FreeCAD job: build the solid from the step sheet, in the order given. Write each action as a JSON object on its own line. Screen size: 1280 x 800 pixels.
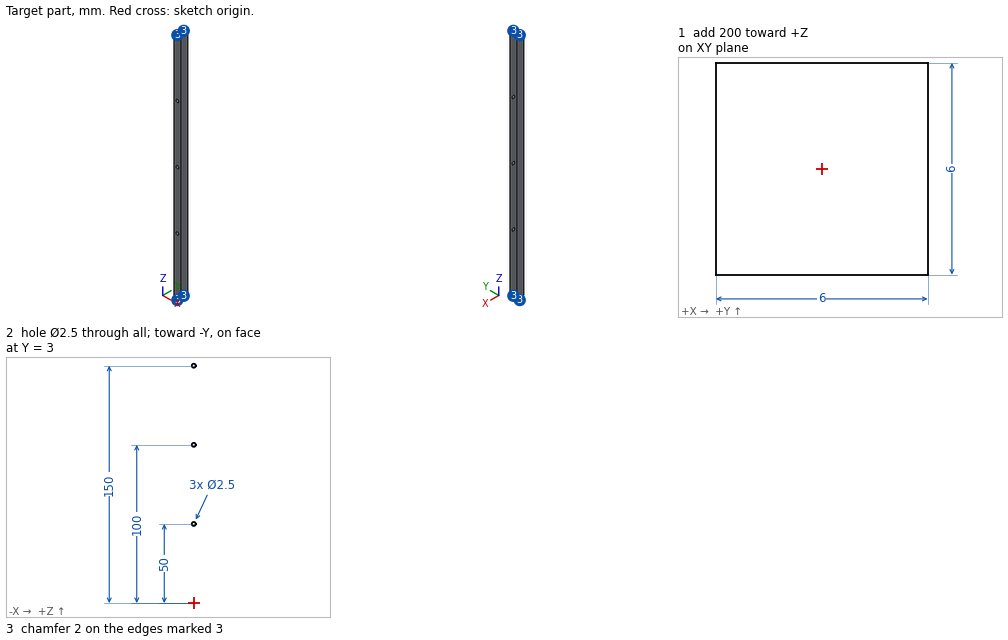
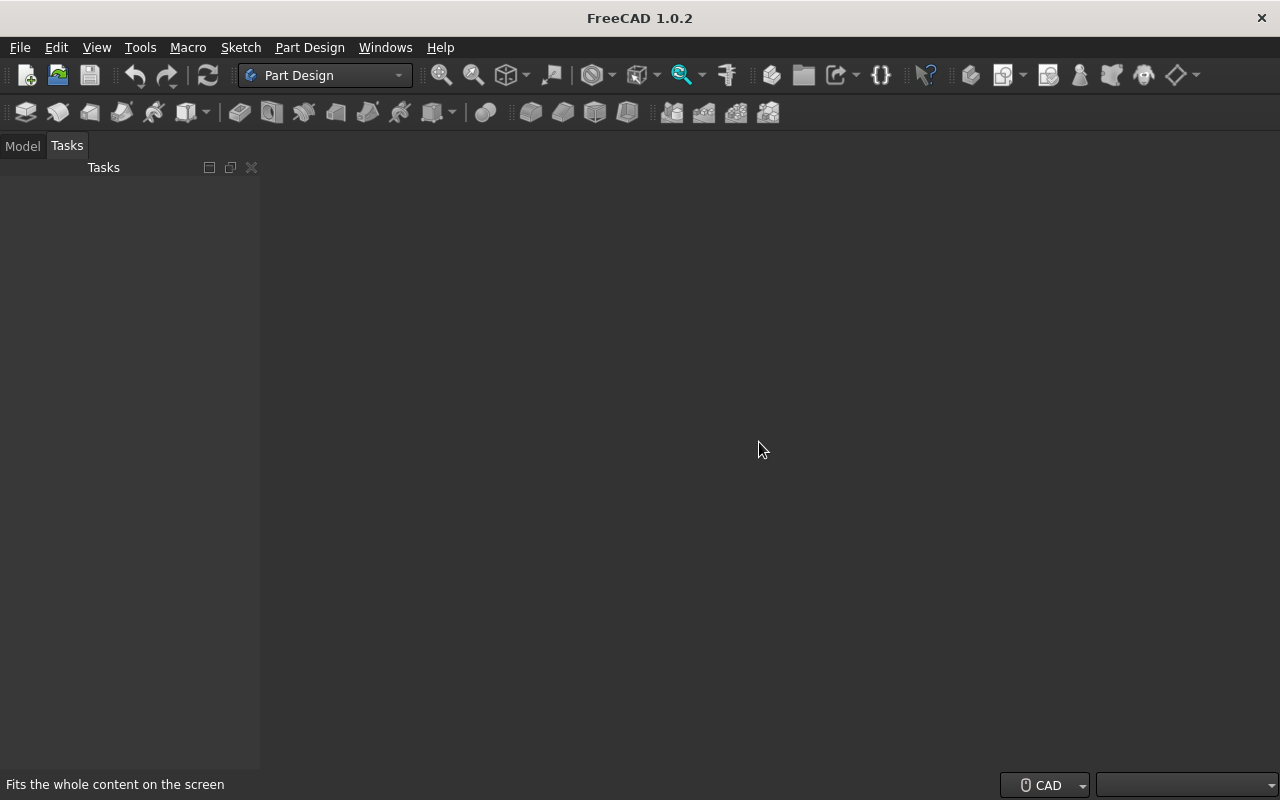
{"action": "left_click", "coordinate": [26, 76]}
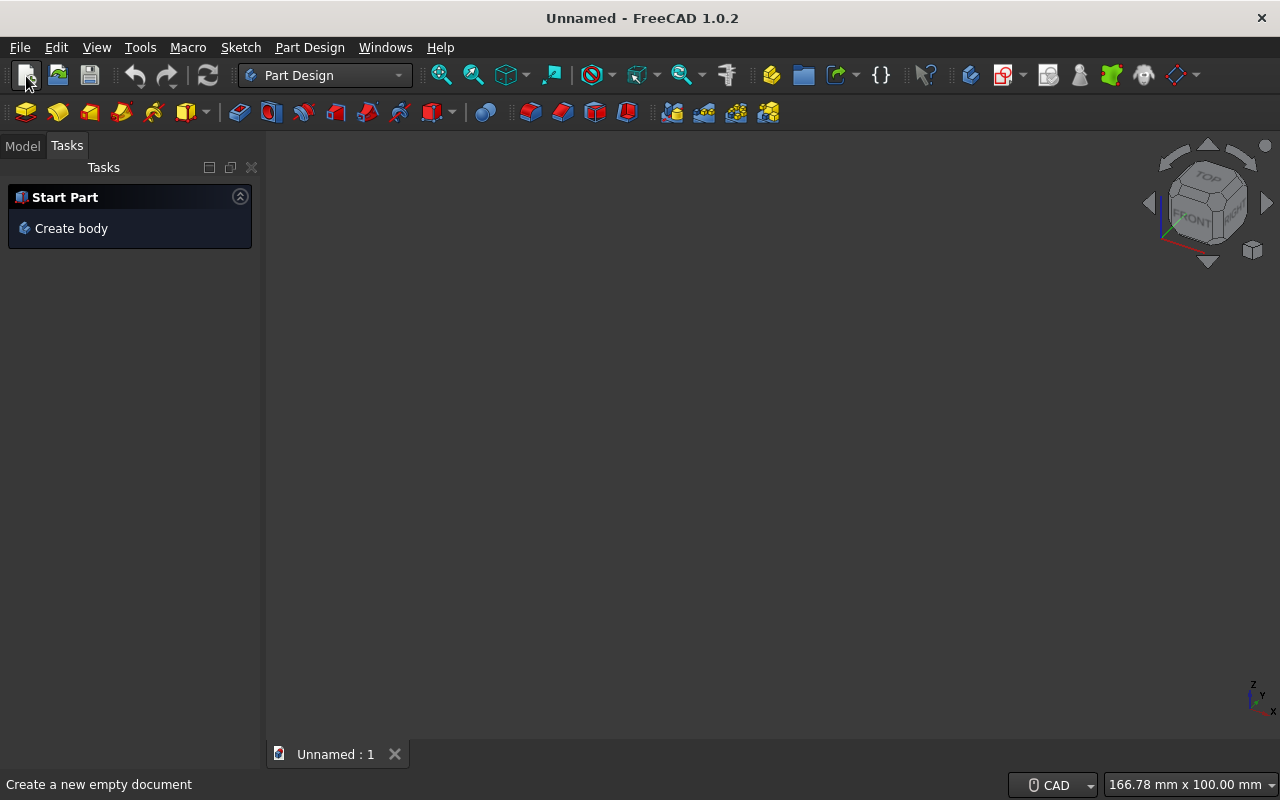
{"action": "left_click", "coordinate": [1004, 76]}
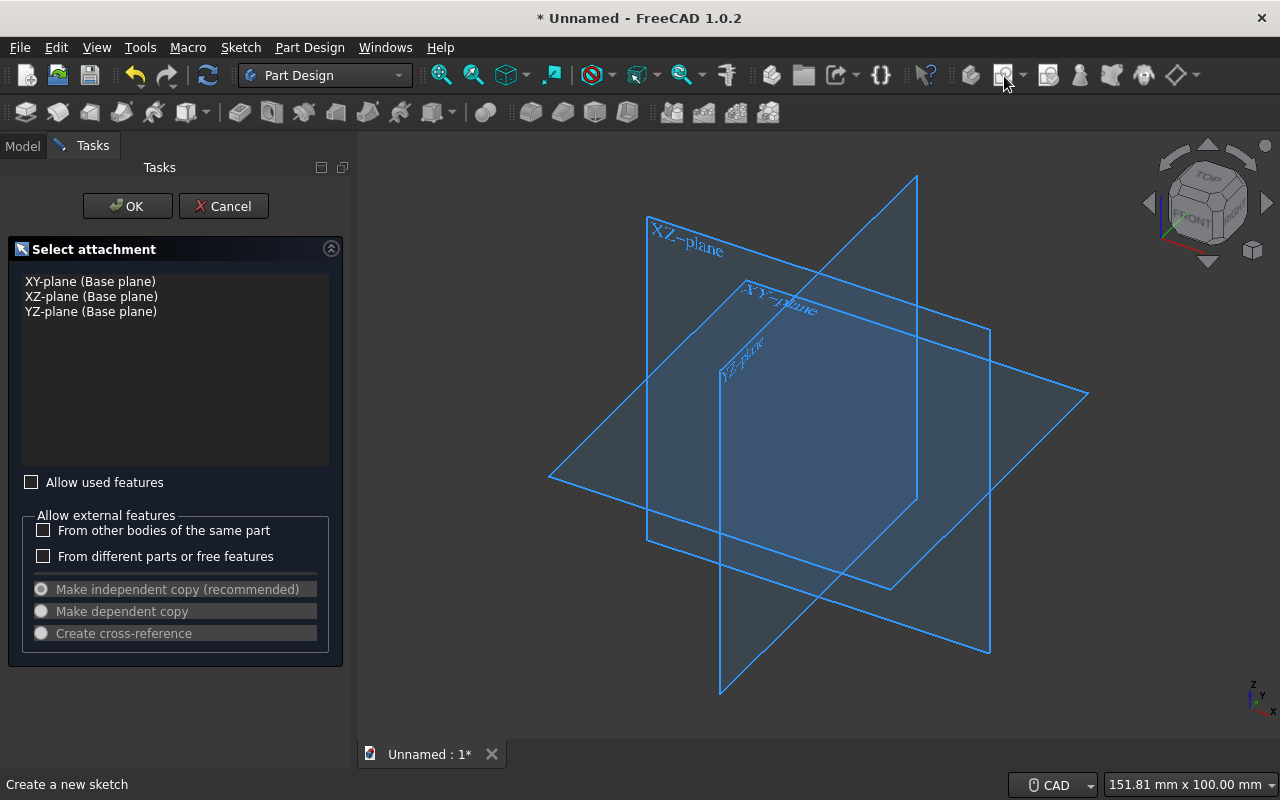
{"action": "left_click", "coordinate": [82, 282]}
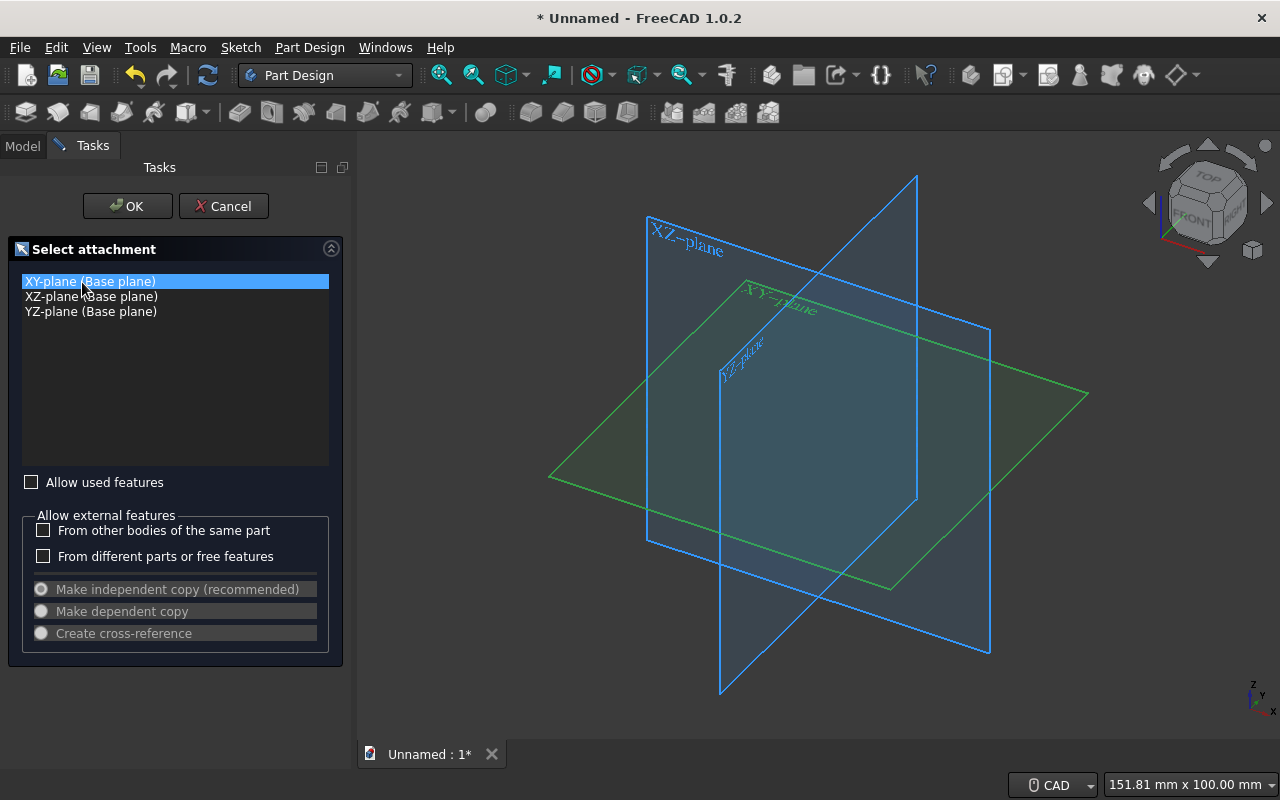
{"action": "left_click", "coordinate": [128, 206]}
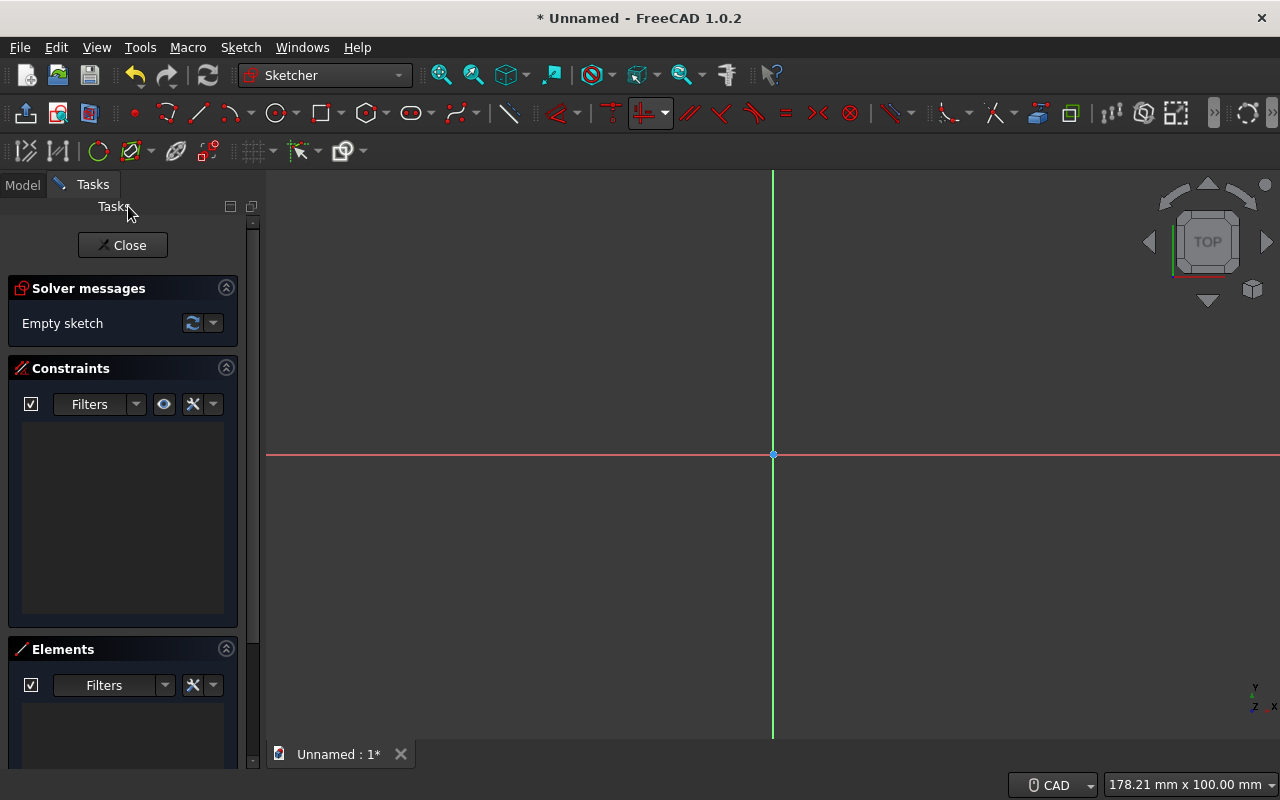
{"action": "scroll", "coordinate": [780, 455], "scroll_direction": "up", "scroll_amount": 12}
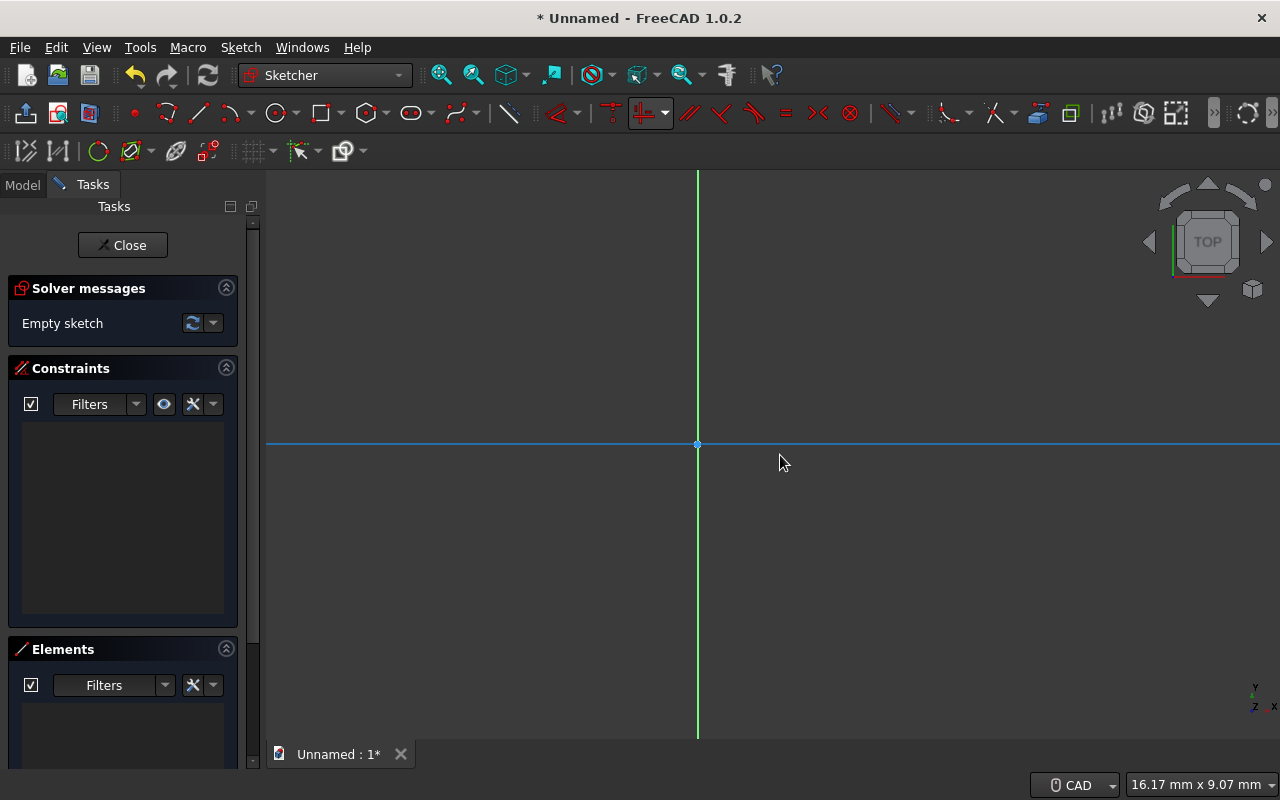
{"action": "left_click", "coordinate": [344, 114]}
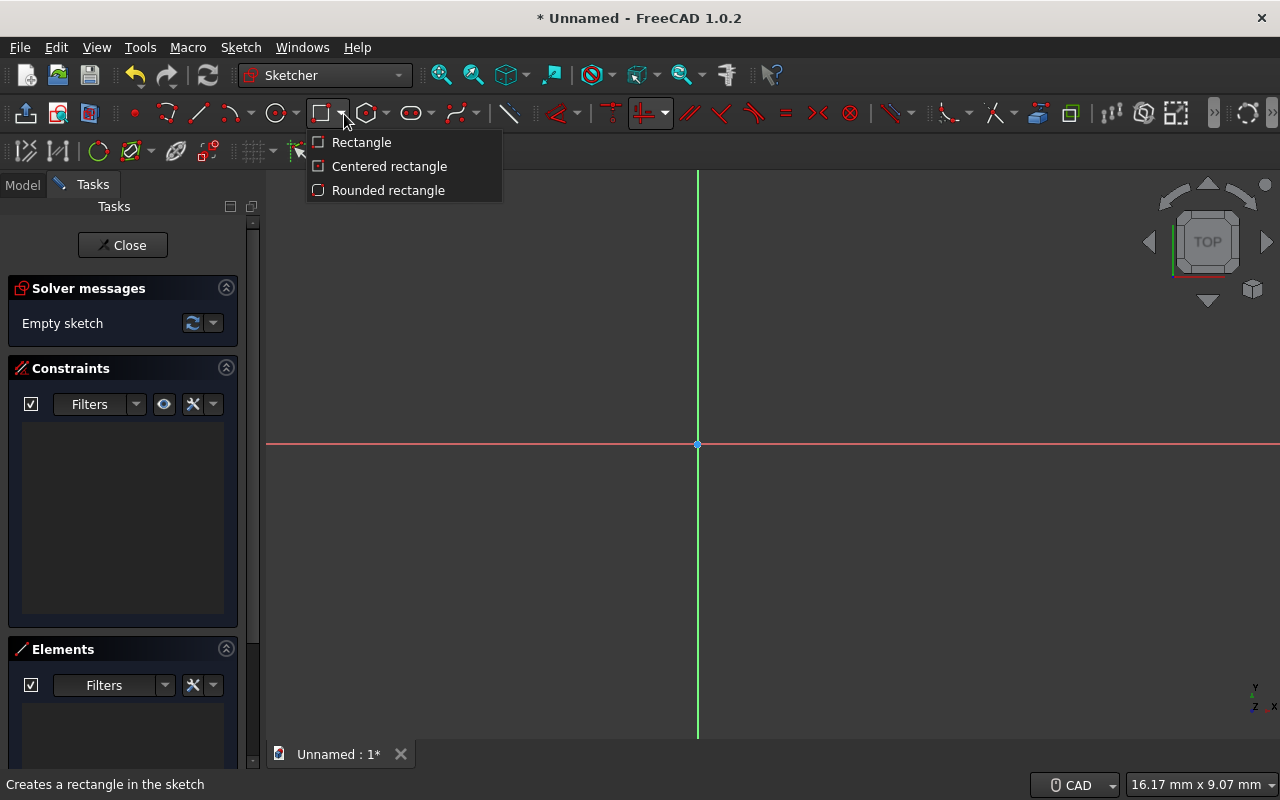
{"action": "left_click", "coordinate": [404, 166]}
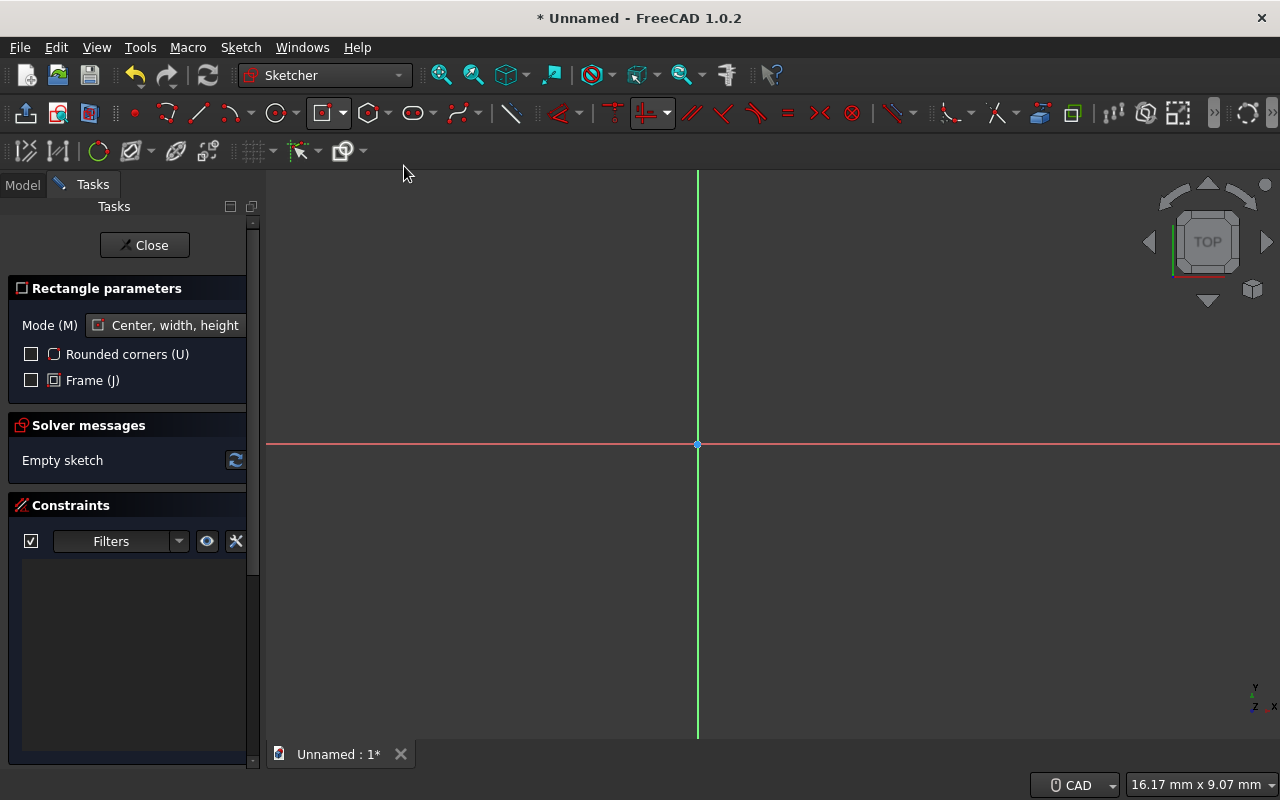
{"action": "left_click", "coordinate": [698, 444]}
{"action": "mouse_move", "coordinate": [886, 256]}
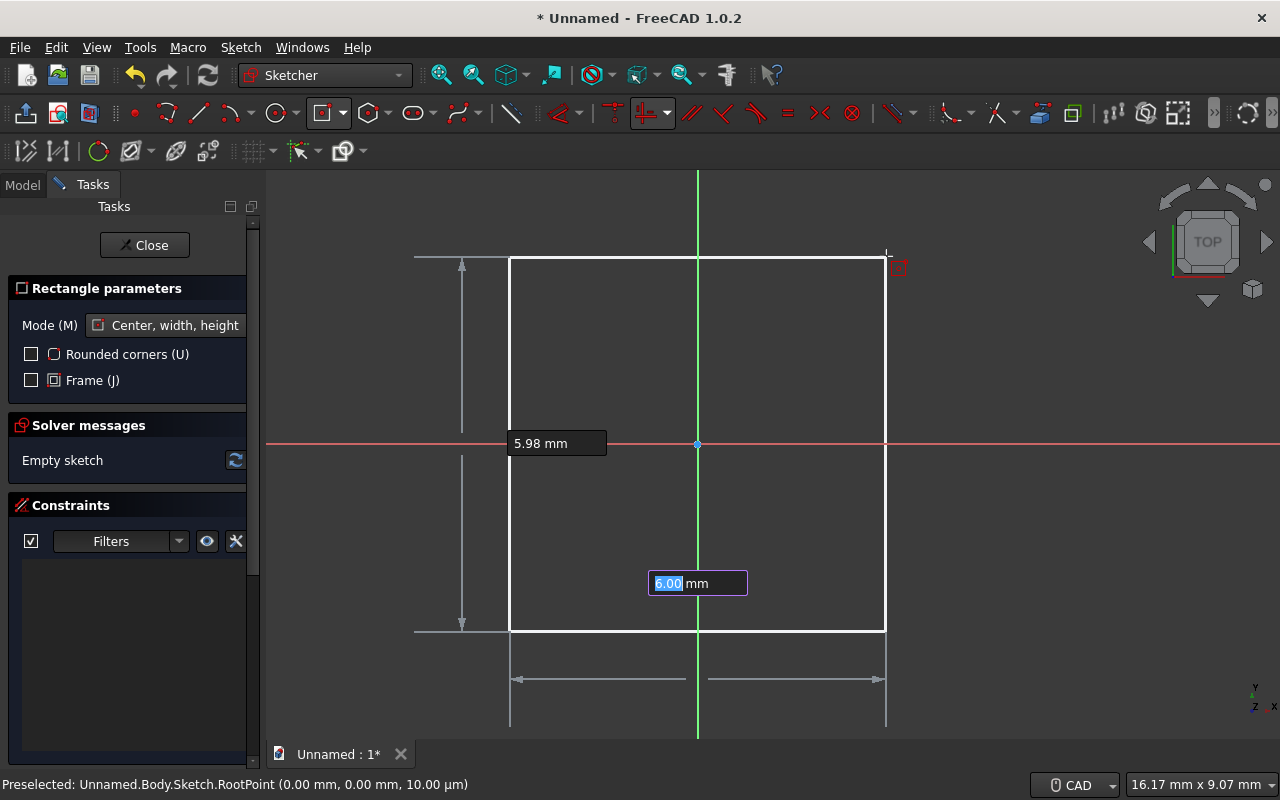
{"action": "type", "text": "6"}
{"action": "key", "text": "Tab"}
{"action": "type", "text": "6"}
{"action": "key", "text": "Return"}
{"action": "key", "text": "Escape"}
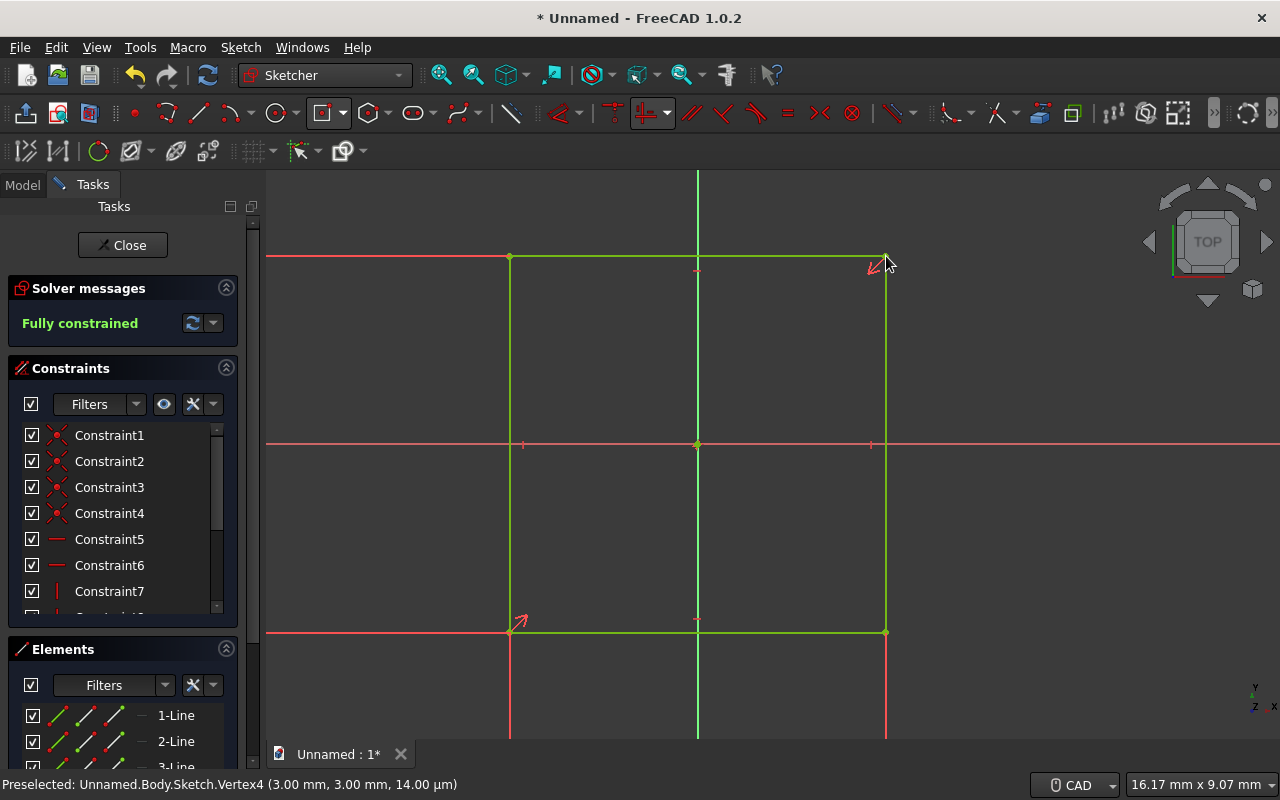
{"action": "left_click", "coordinate": [123, 245]}